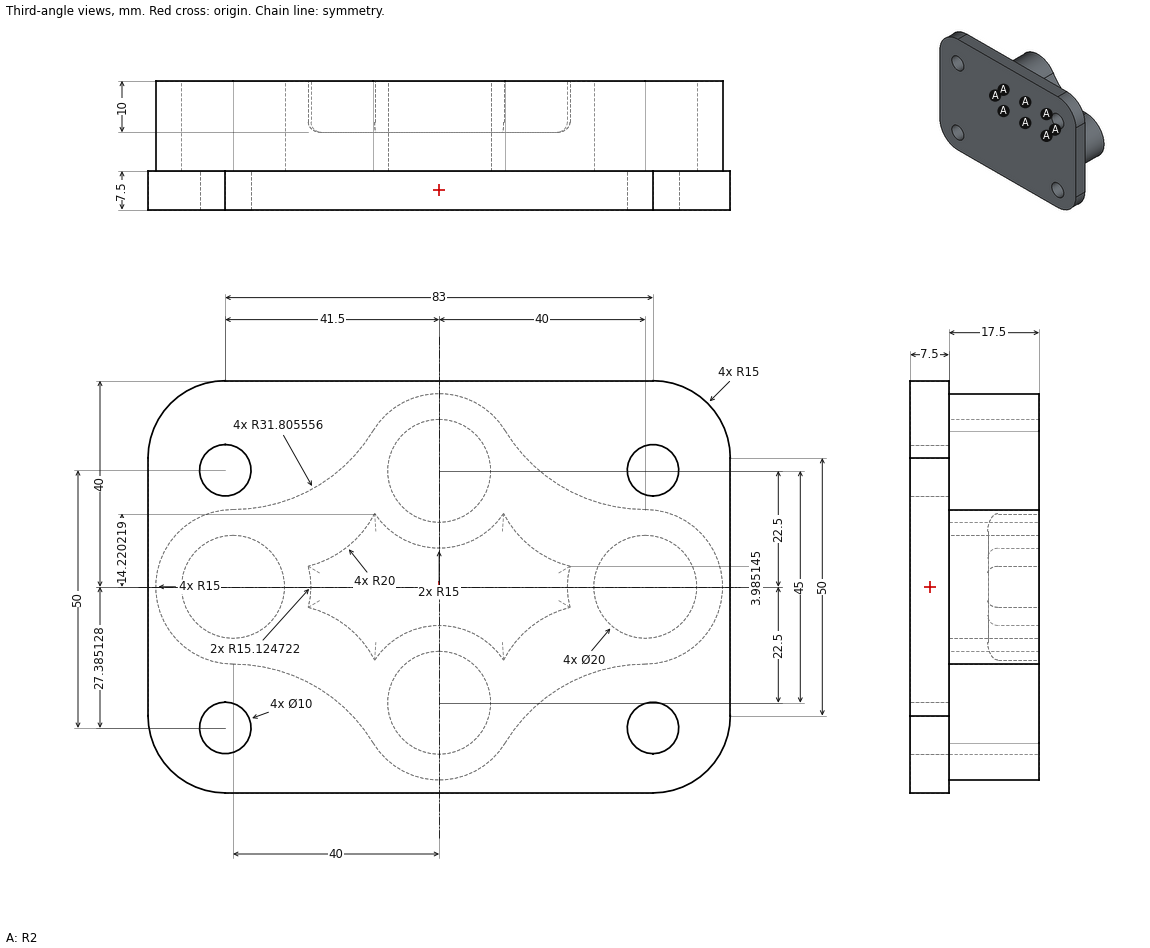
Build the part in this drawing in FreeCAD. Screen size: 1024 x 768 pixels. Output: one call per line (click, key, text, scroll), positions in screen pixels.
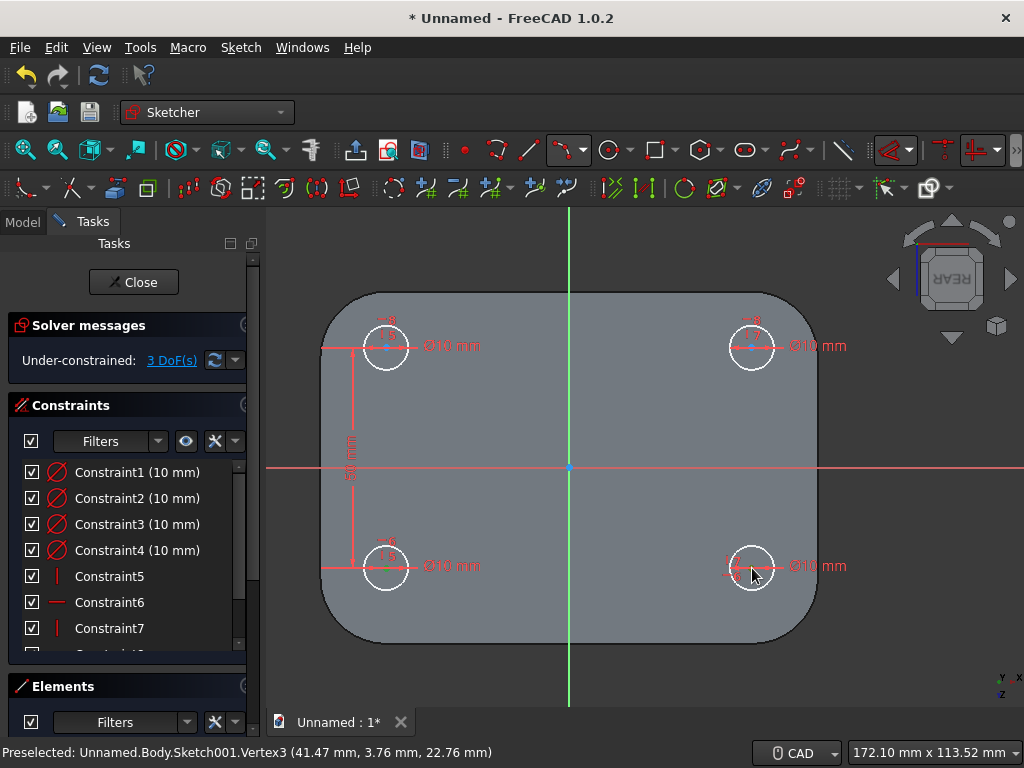
key(l)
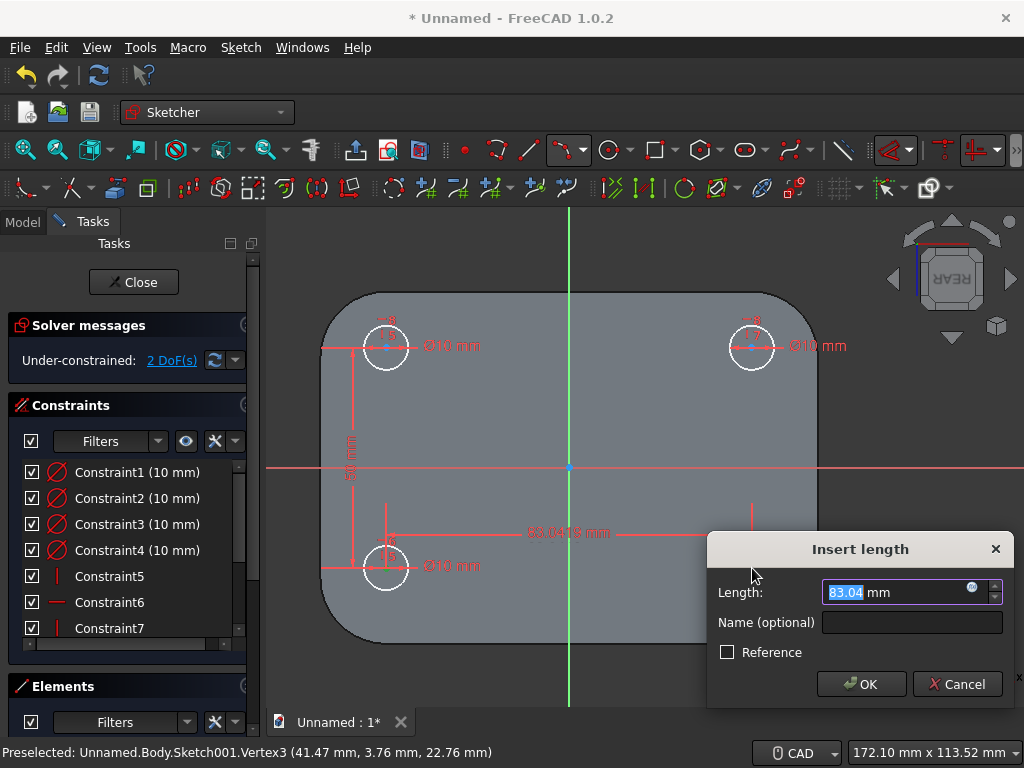
text(83)
key(Return)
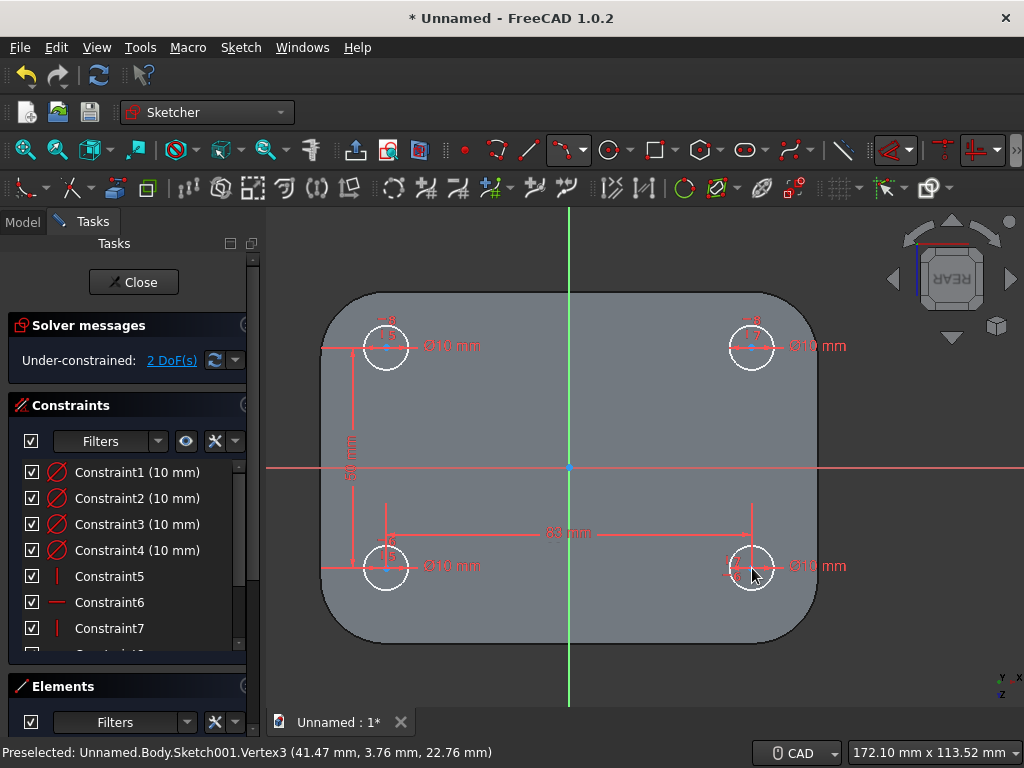
click(386, 348)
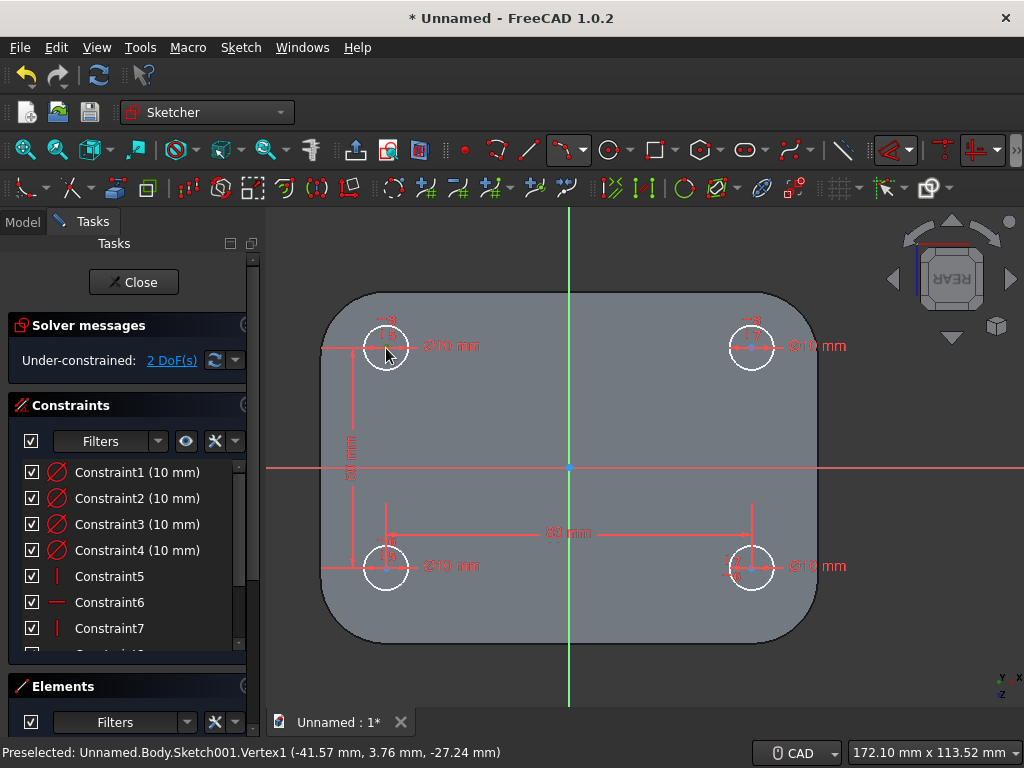
key(l)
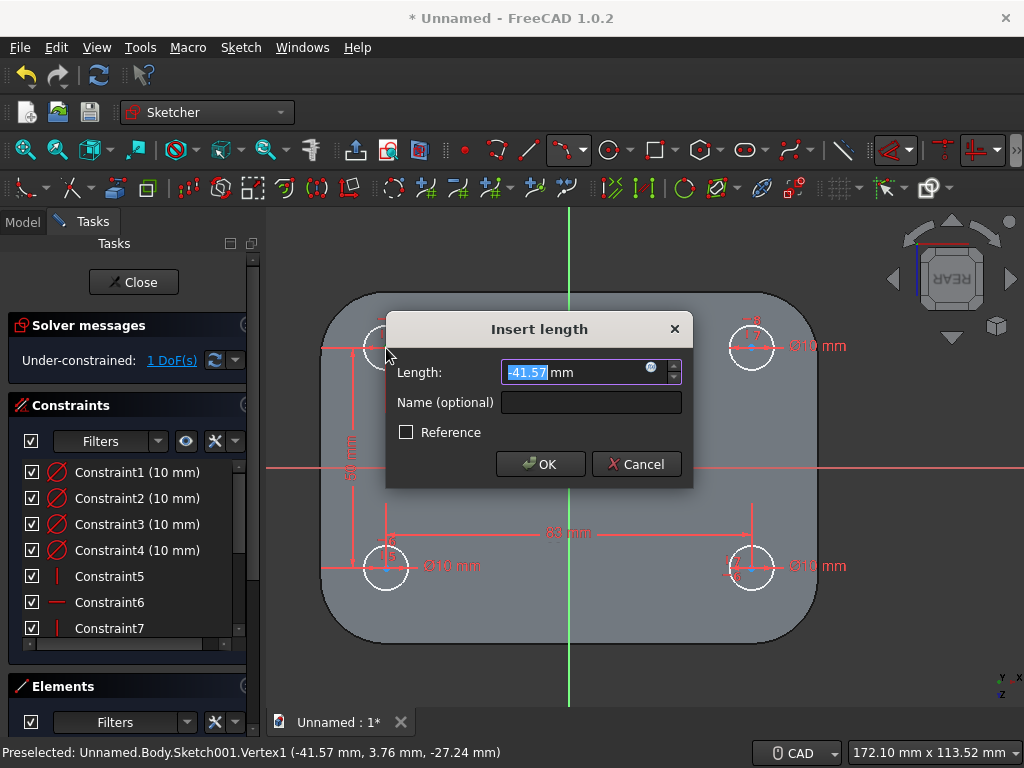
text(-41.5)
key(Return)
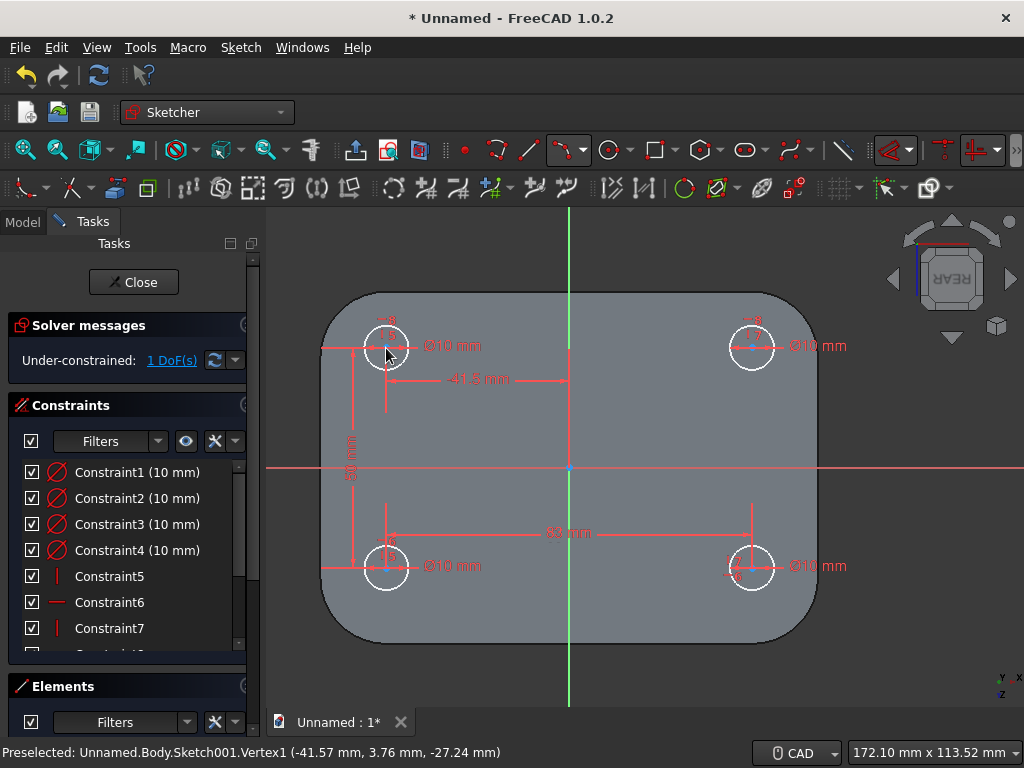
click(386, 348)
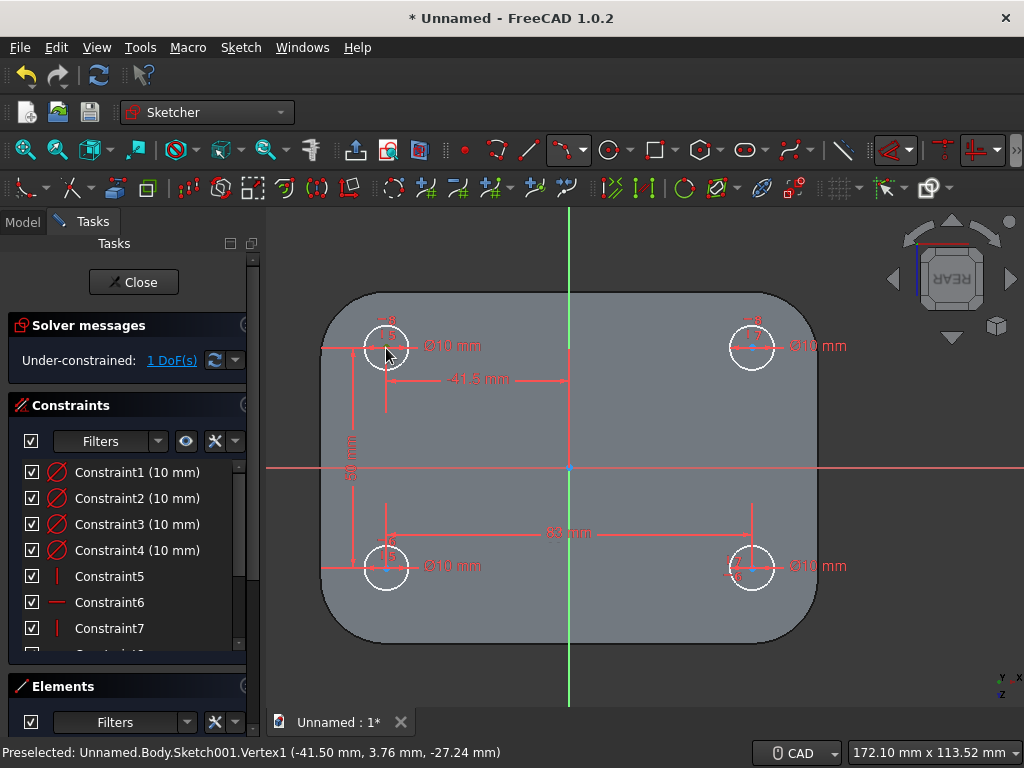
click(912, 150)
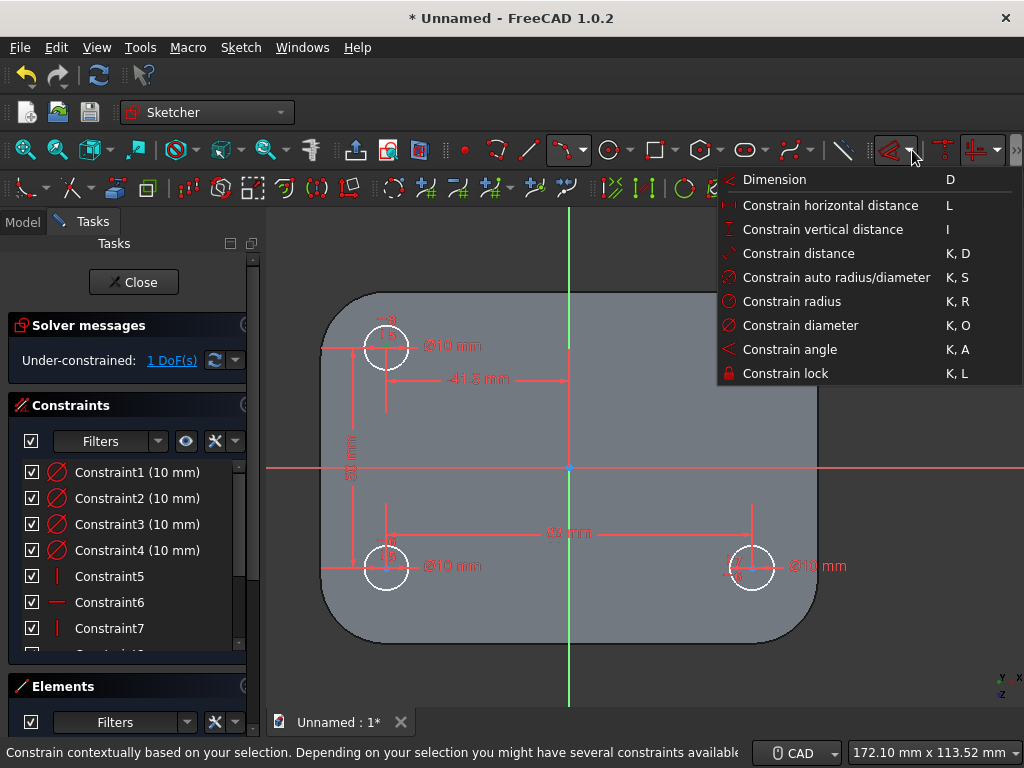
click(870, 229)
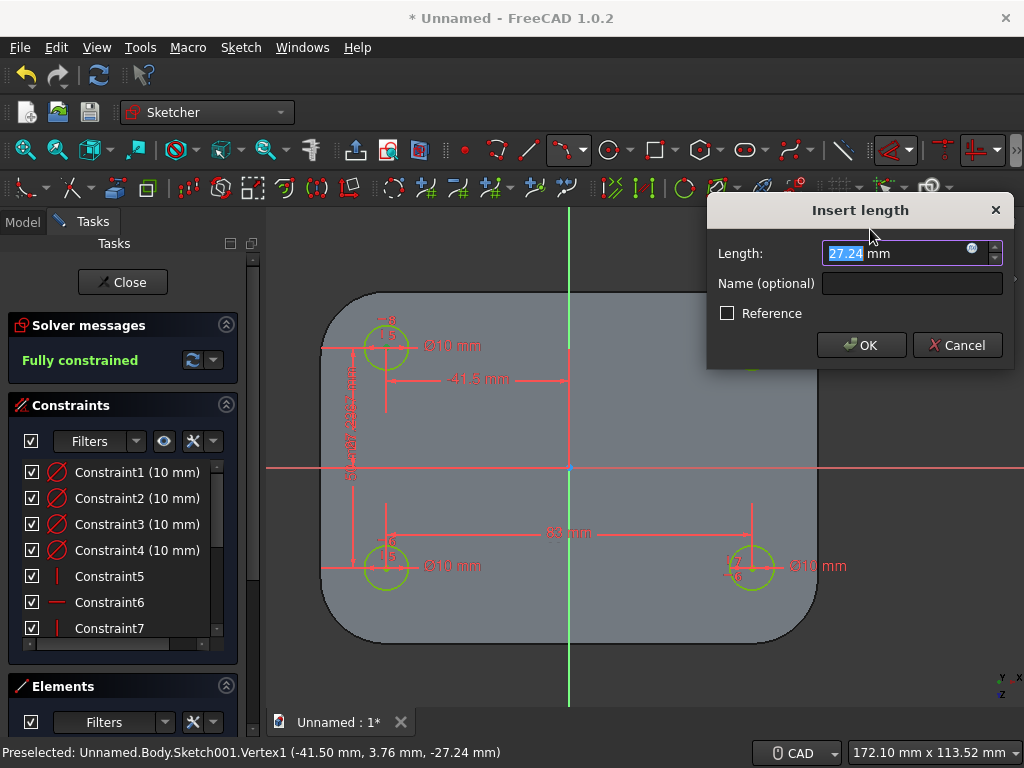
text(27.385128)
key(Return)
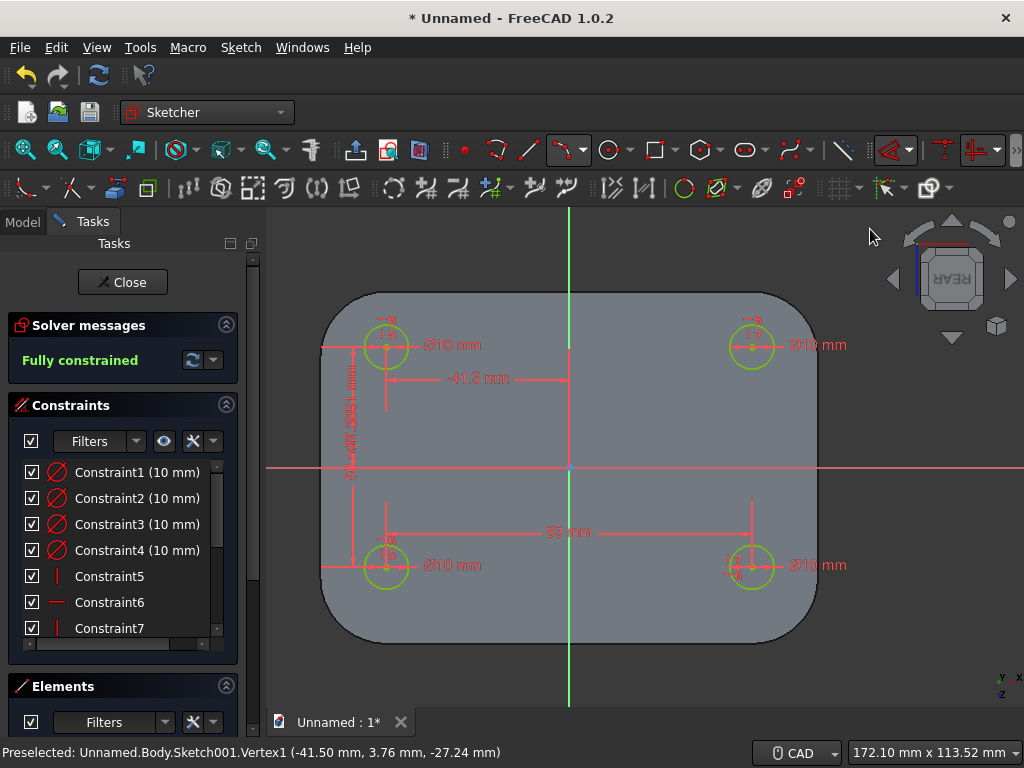
click(123, 282)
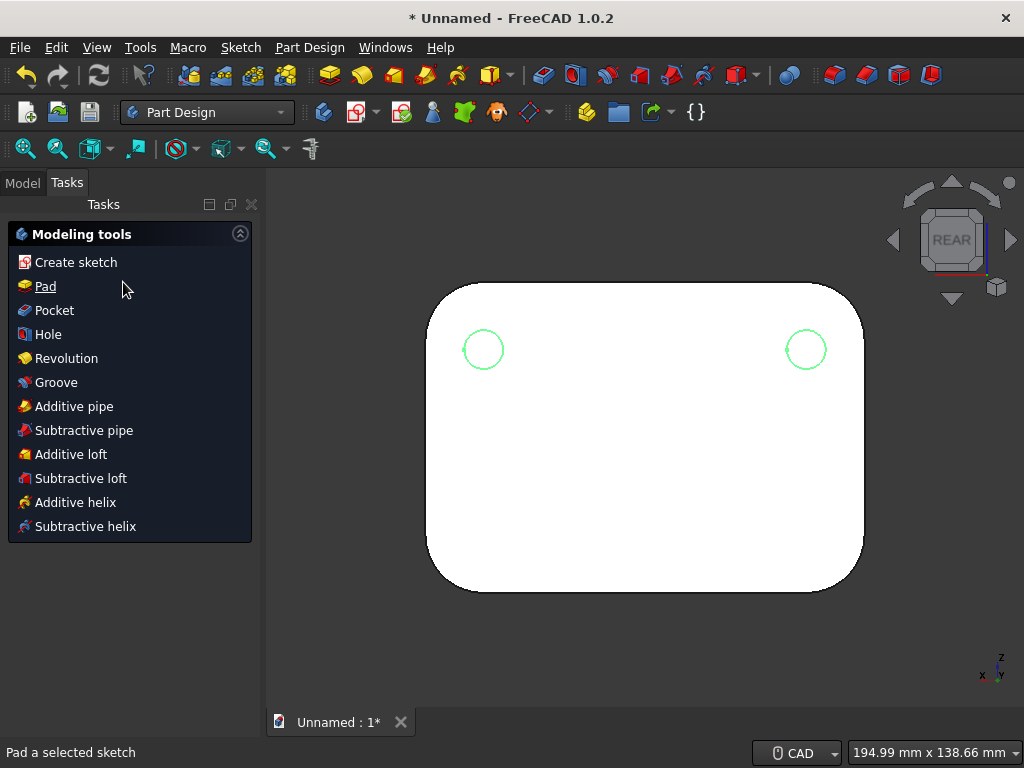
click(544, 76)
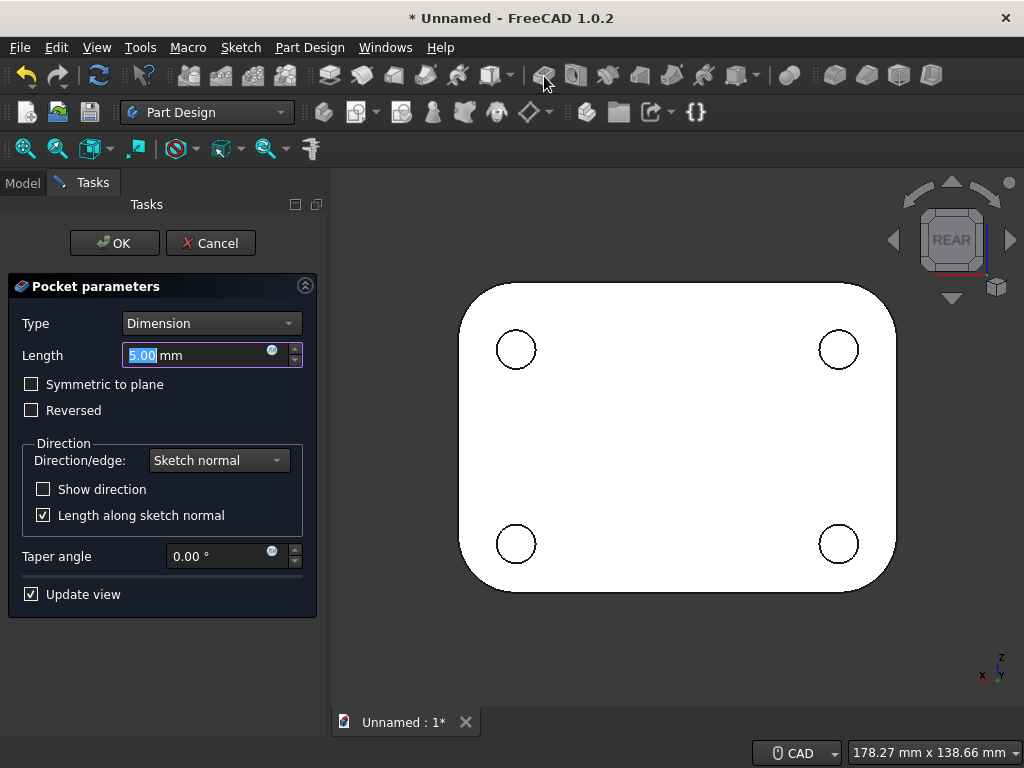
text(7.5)
key(Tab)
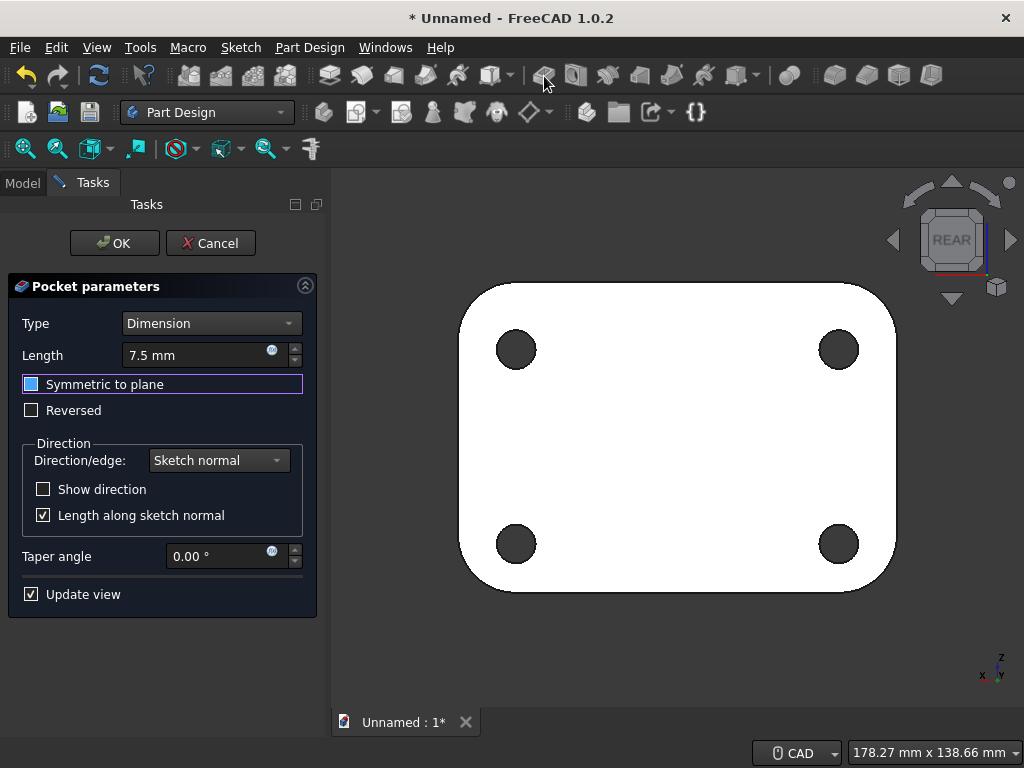
click(115, 243)